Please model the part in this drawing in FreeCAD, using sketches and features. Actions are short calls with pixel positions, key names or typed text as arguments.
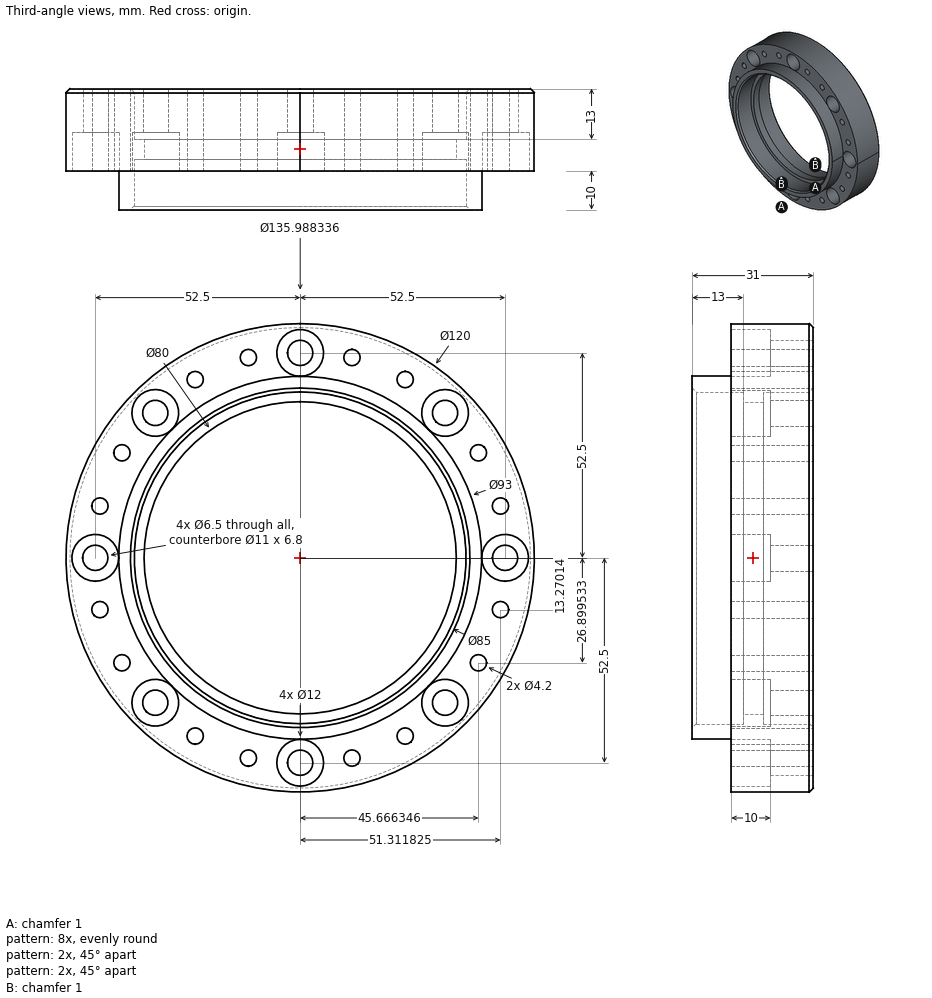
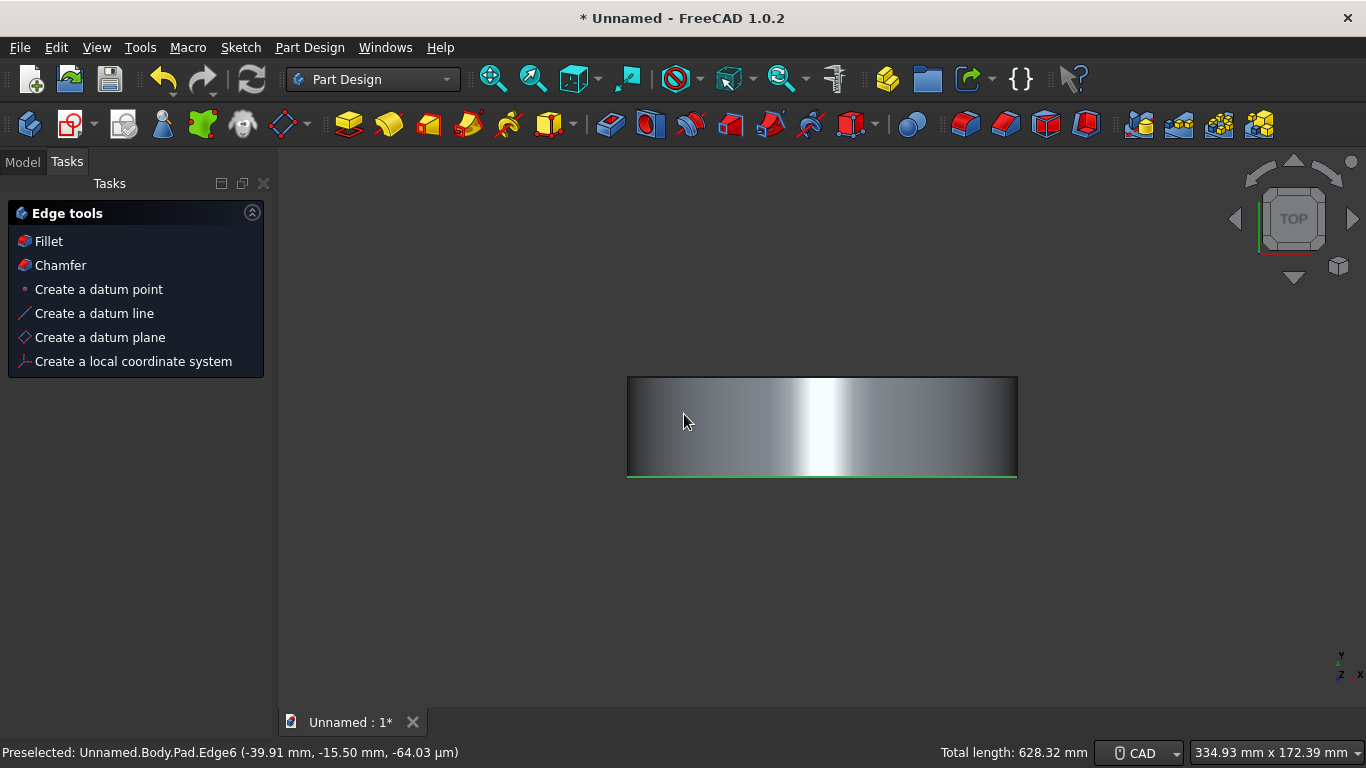
click(494, 80)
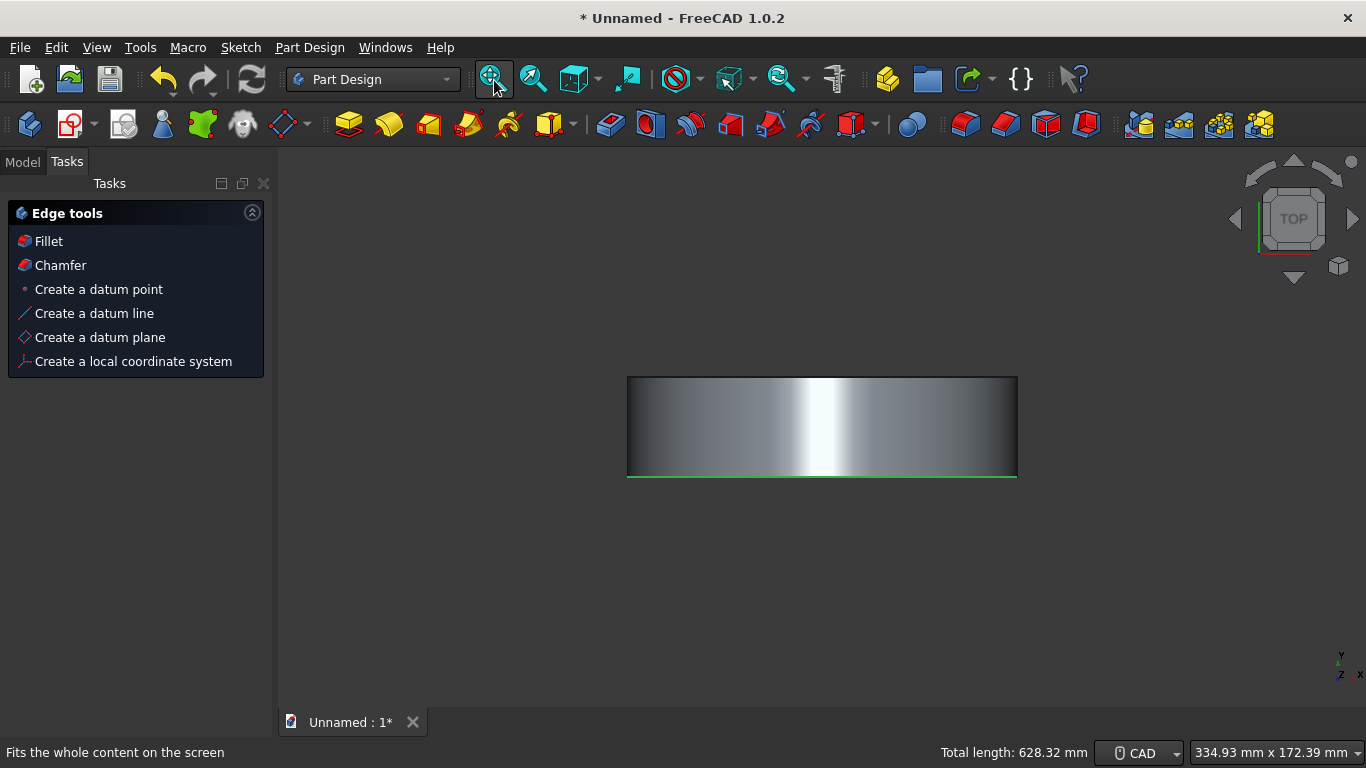
click(664, 376, ctrl)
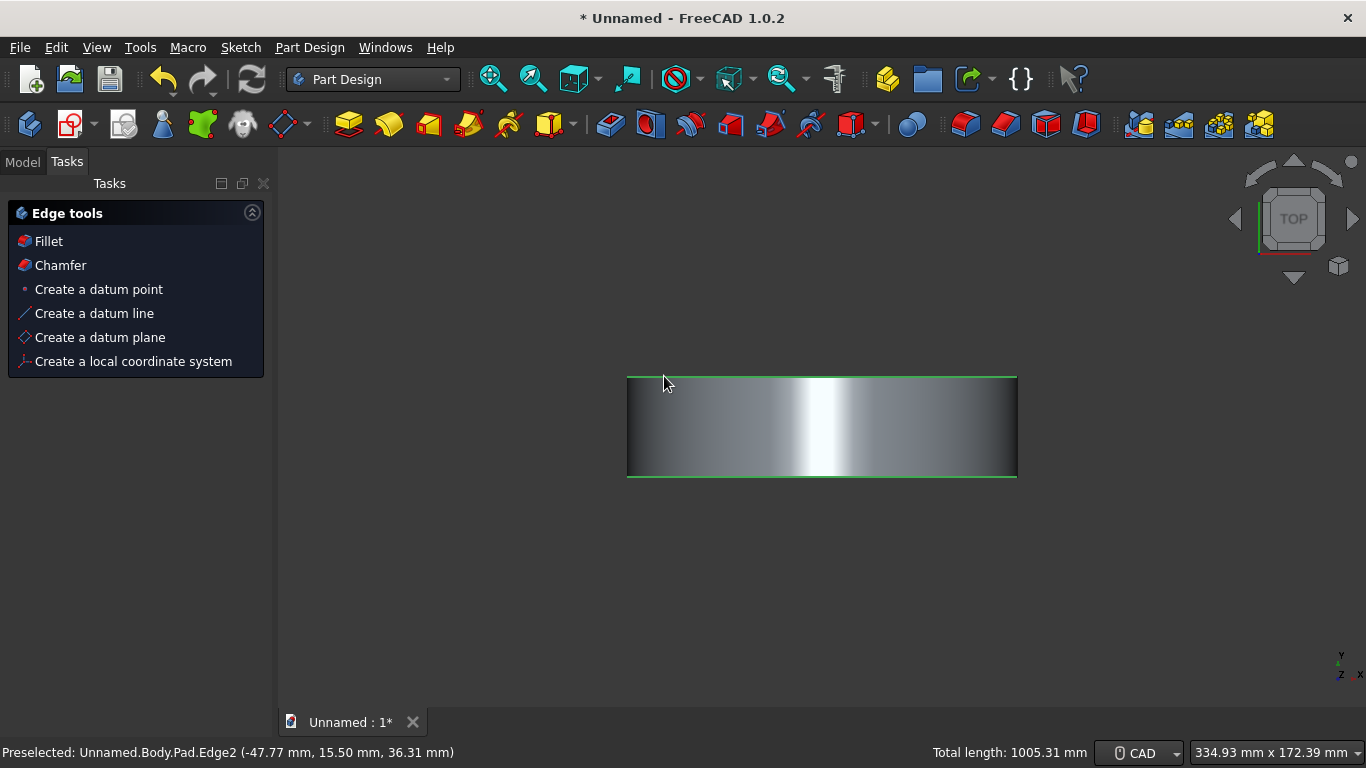
key(1)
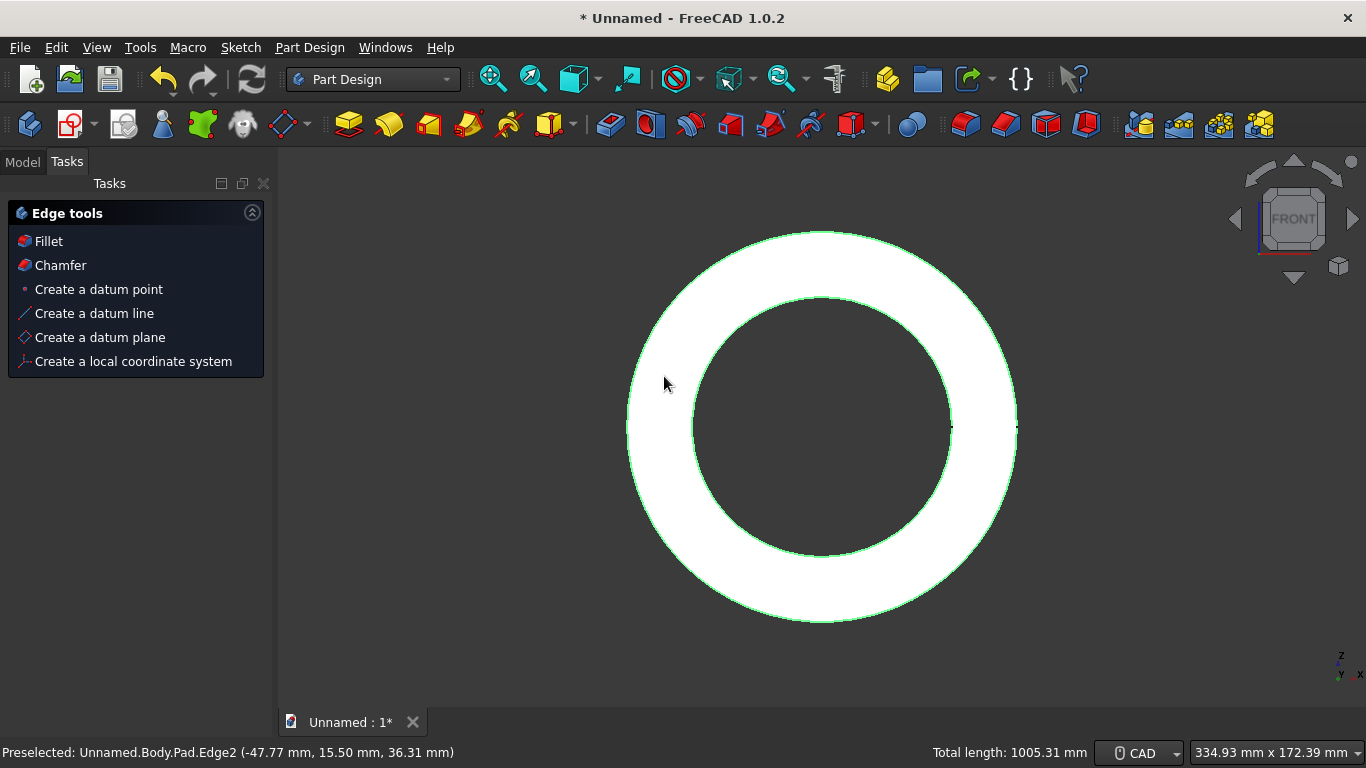
key(3)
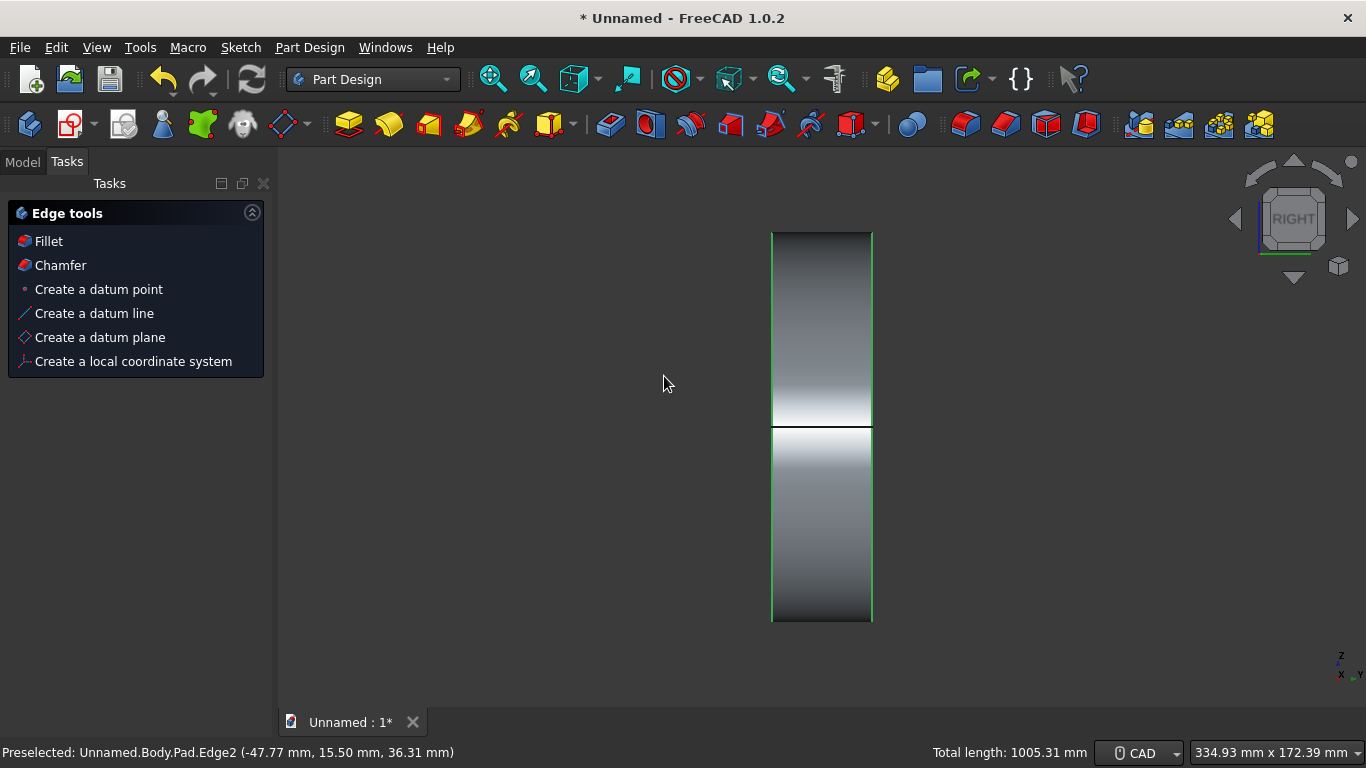
key(5)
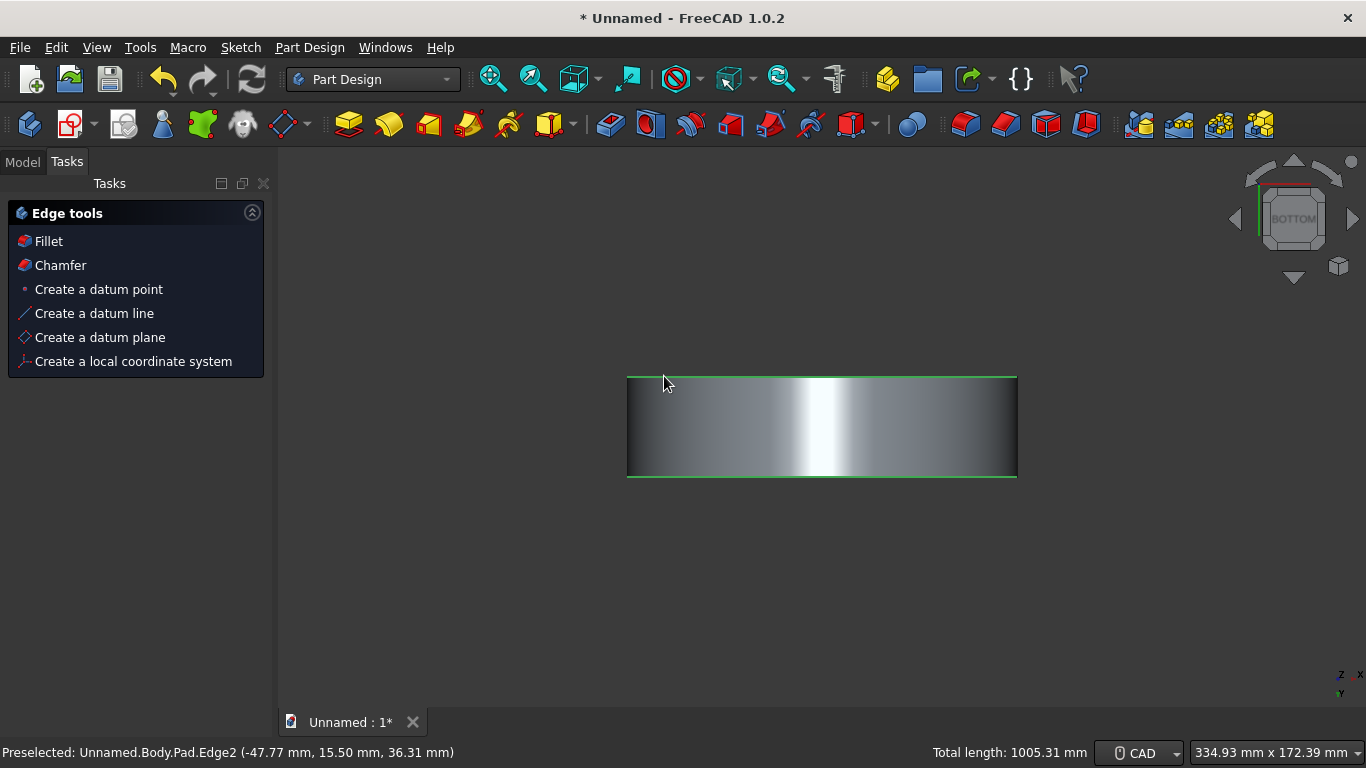
click(494, 80)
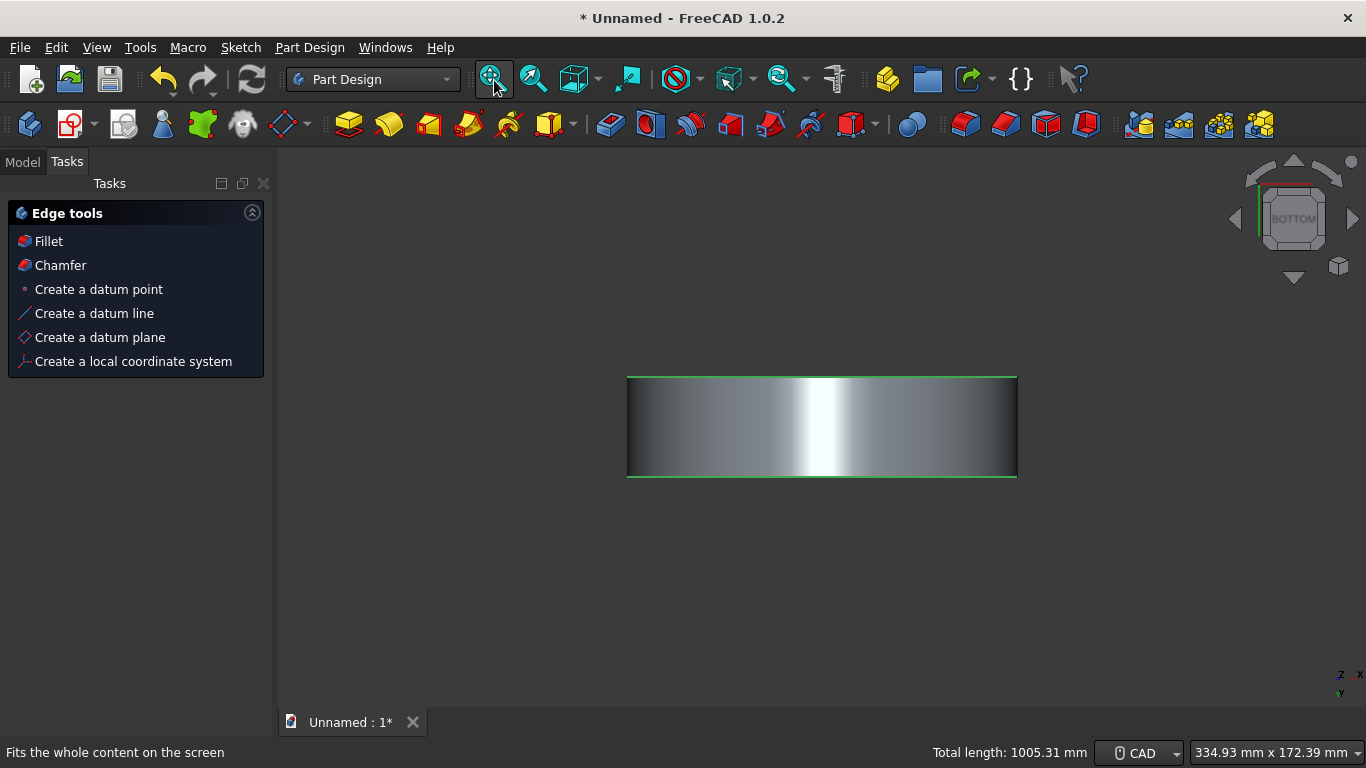
key(4)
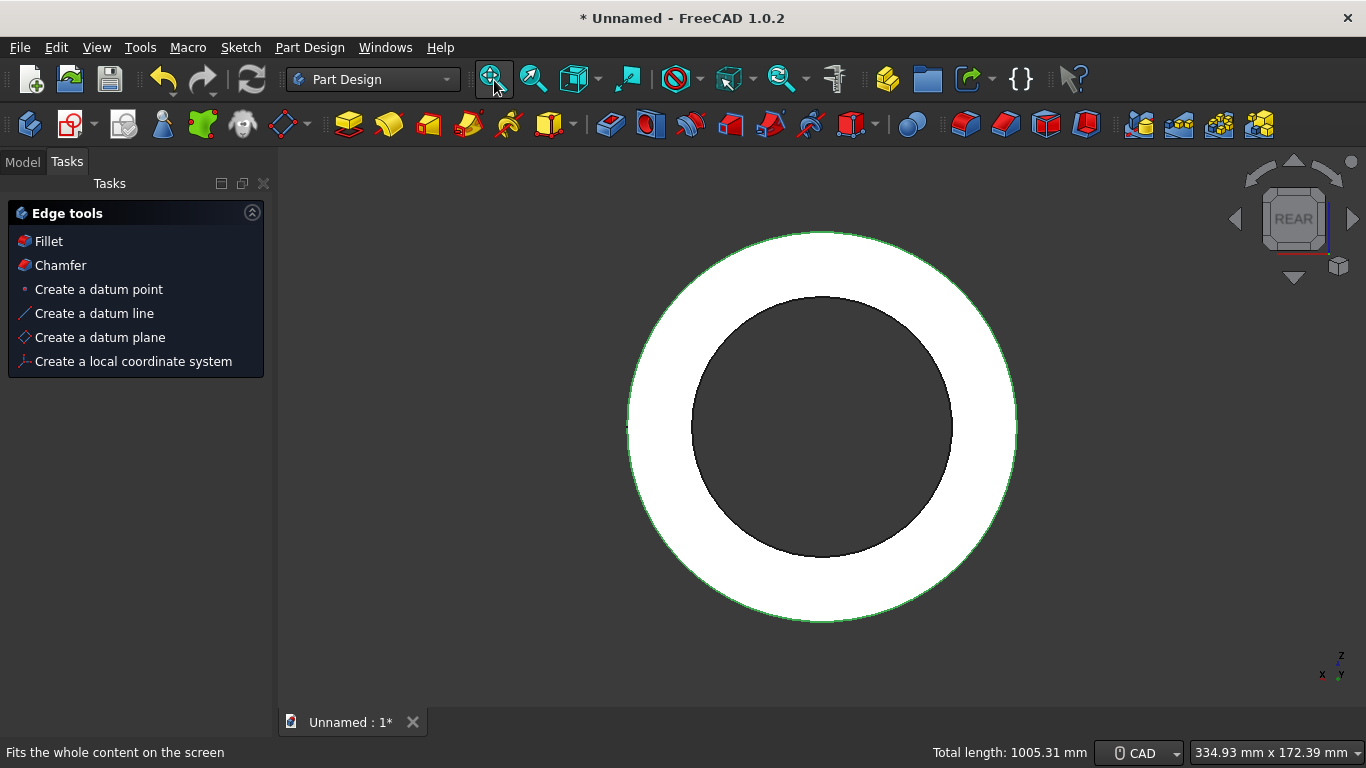
click(952, 426, ctrl)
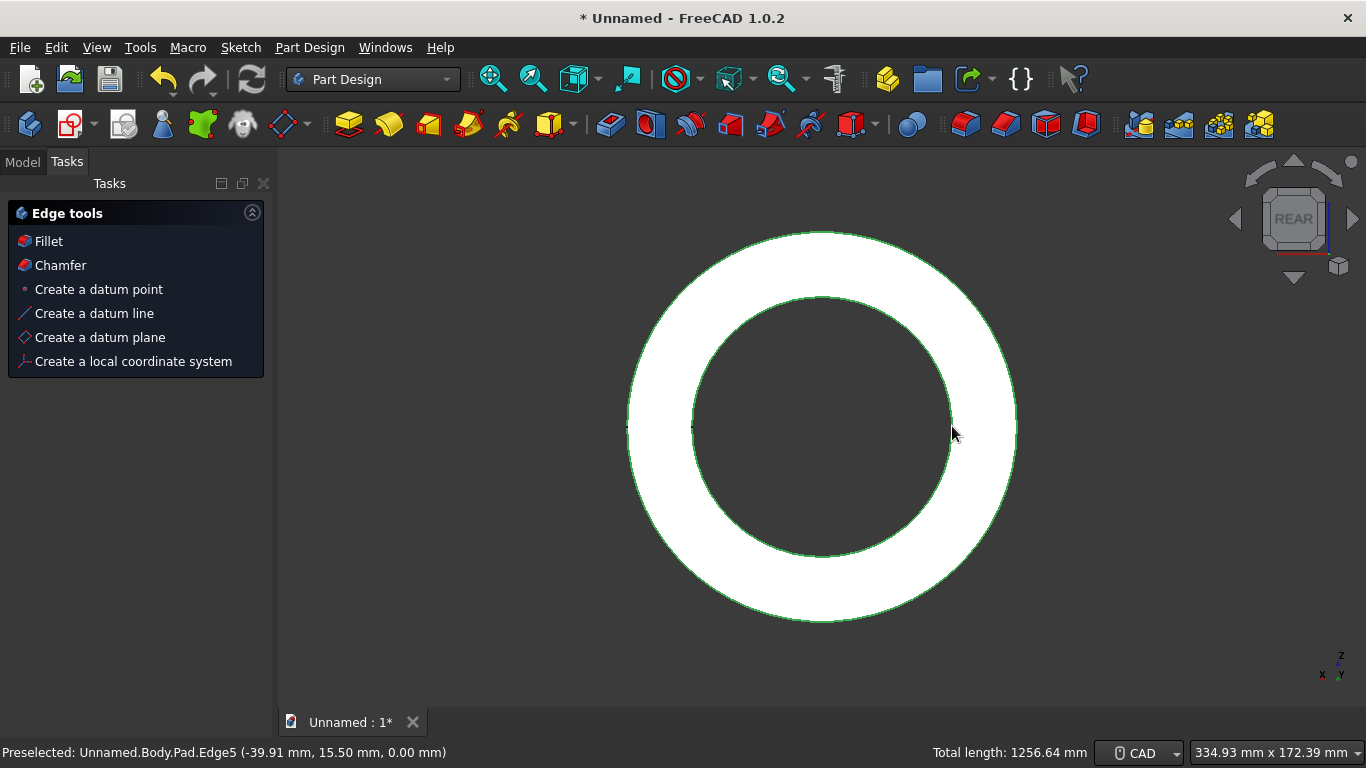
click(1006, 124)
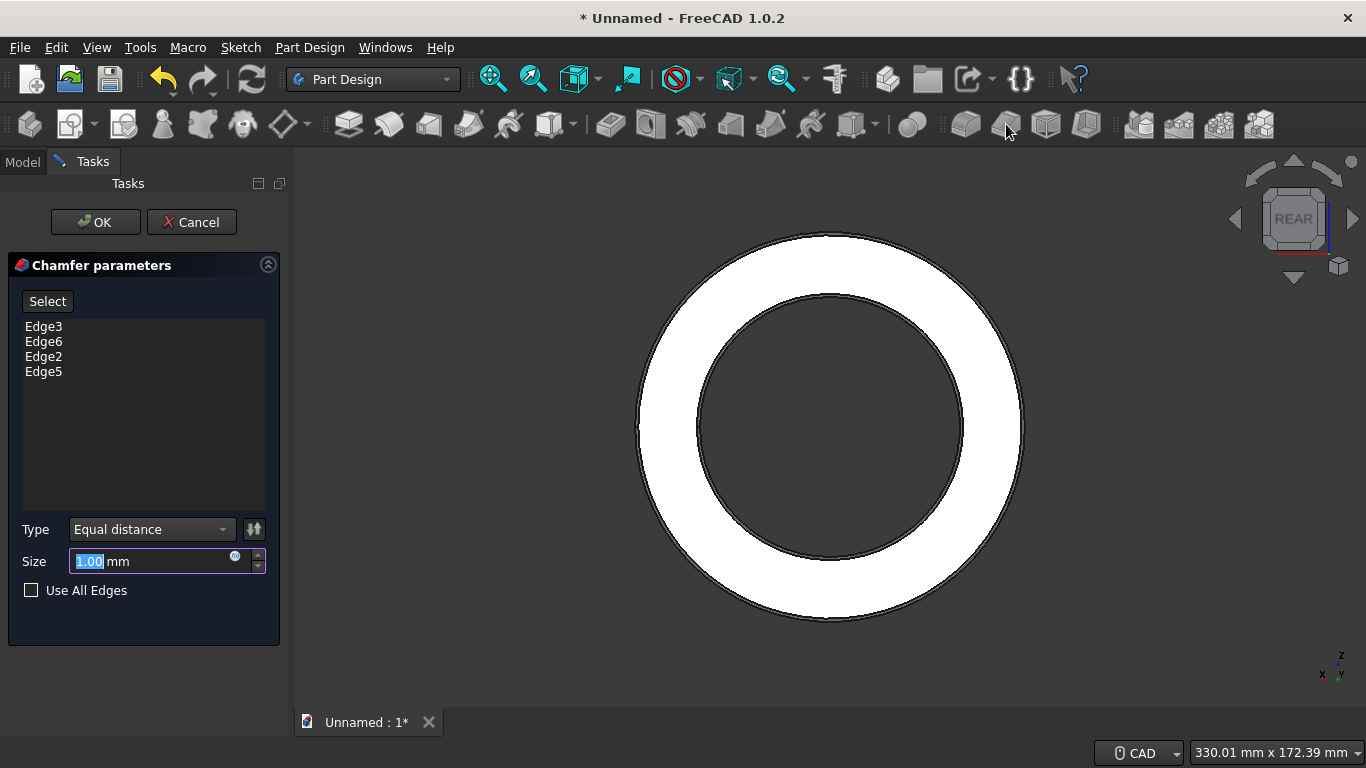
text(1)
key(Tab)